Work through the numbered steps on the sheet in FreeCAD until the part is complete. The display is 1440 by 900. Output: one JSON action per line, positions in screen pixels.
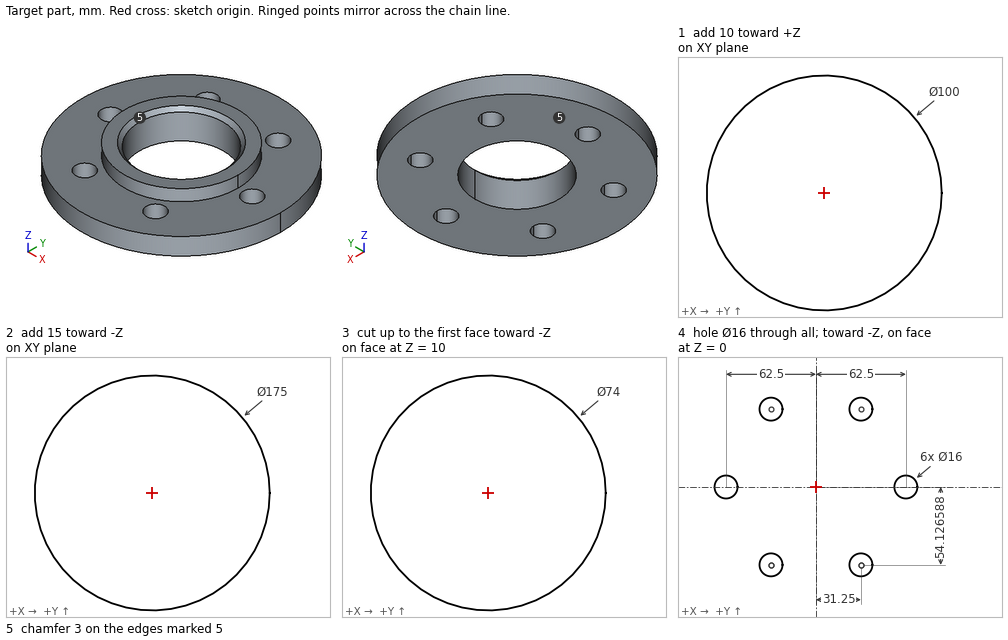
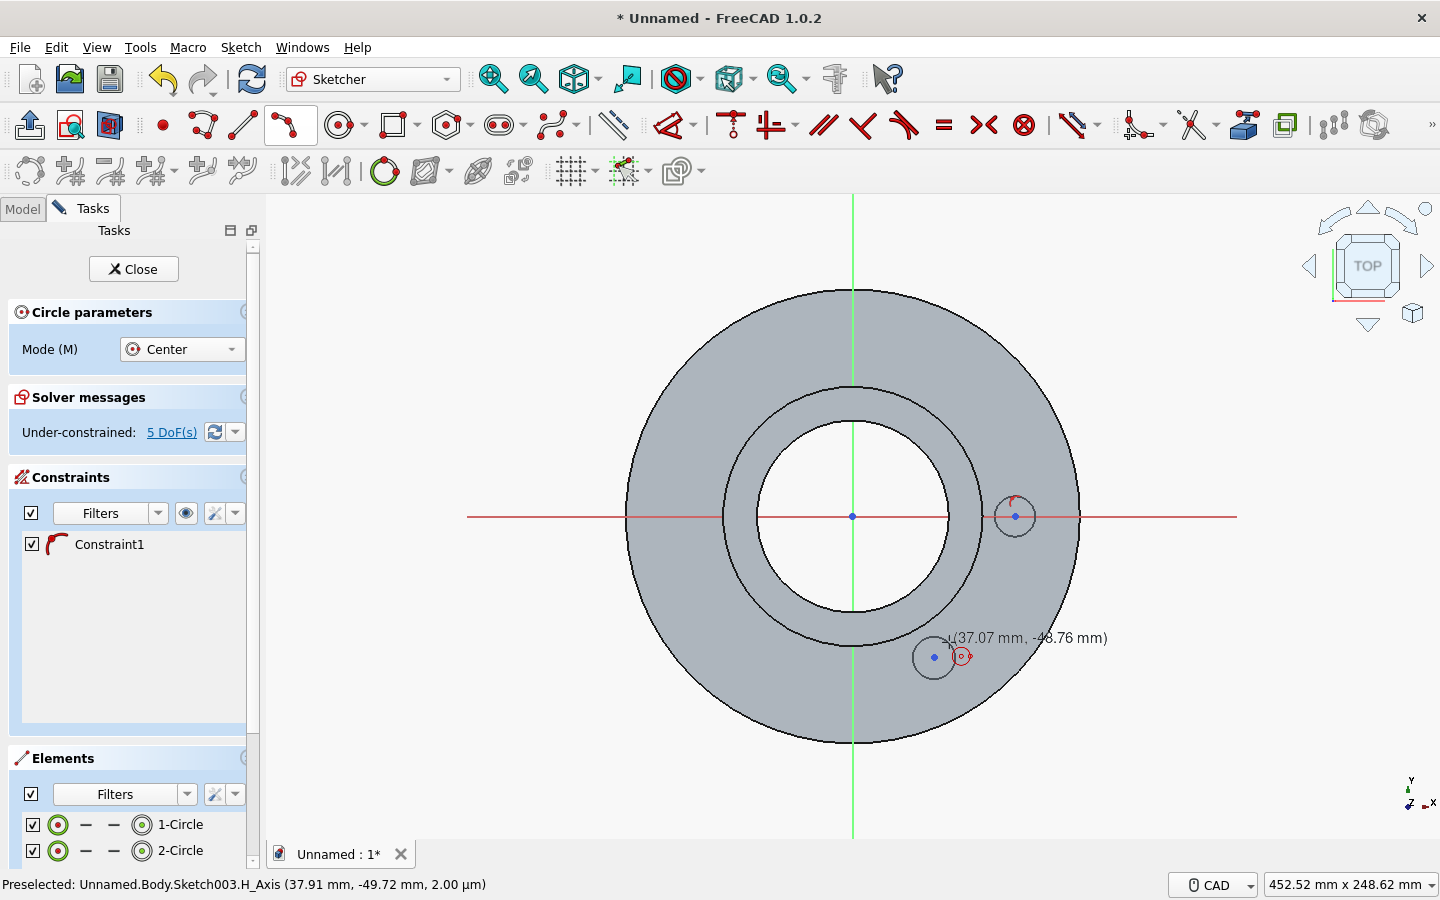
{"action": "left_click", "coordinate": [772, 657]}
{"action": "left_click", "coordinate": [786, 642]}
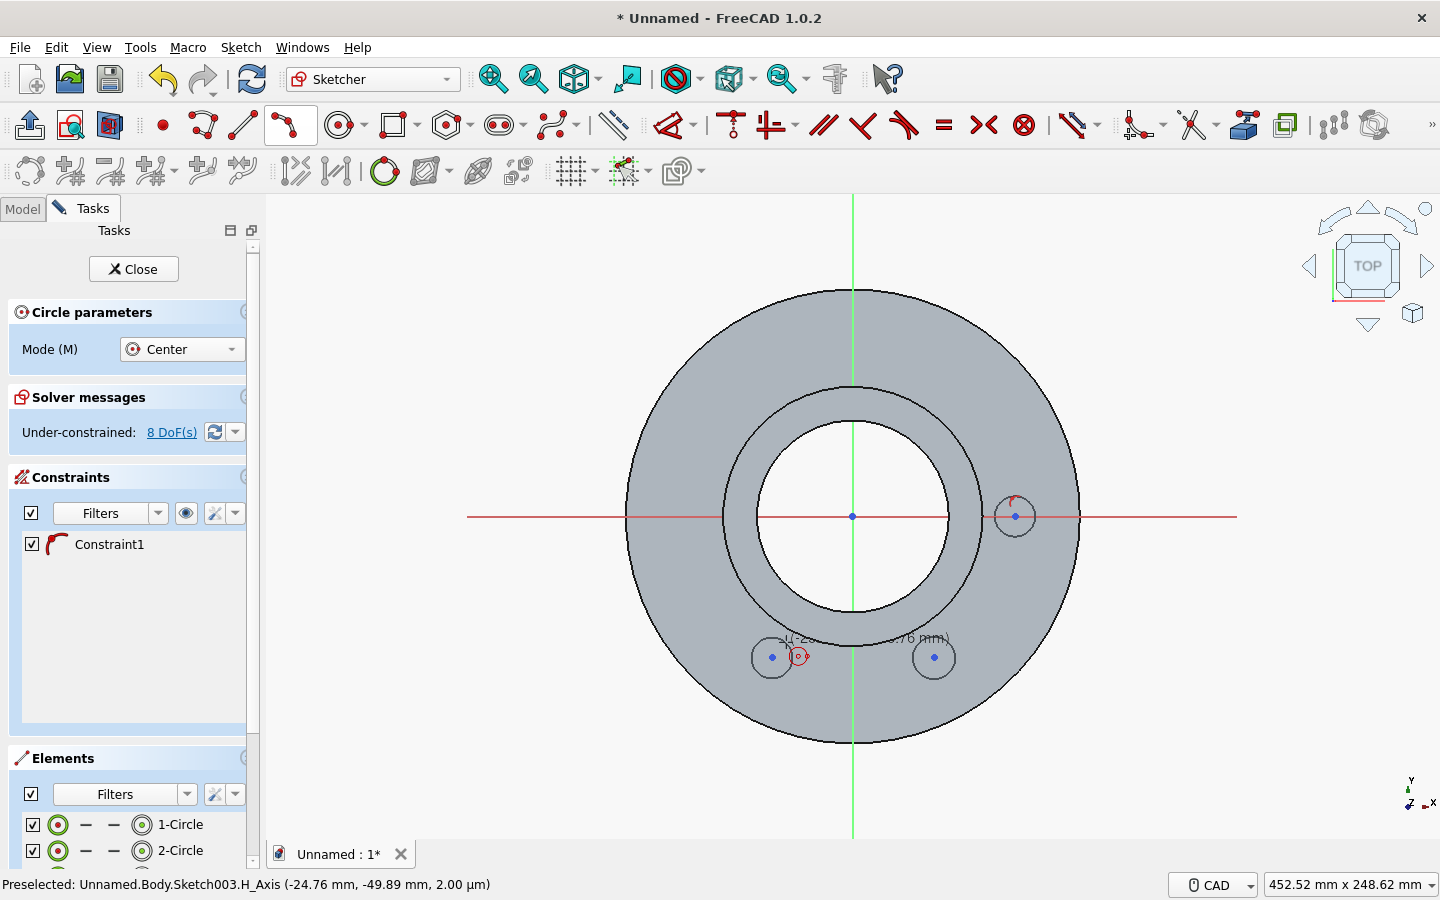
{"action": "left_click", "coordinate": [691, 516]}
{"action": "left_click", "coordinate": [705, 502]}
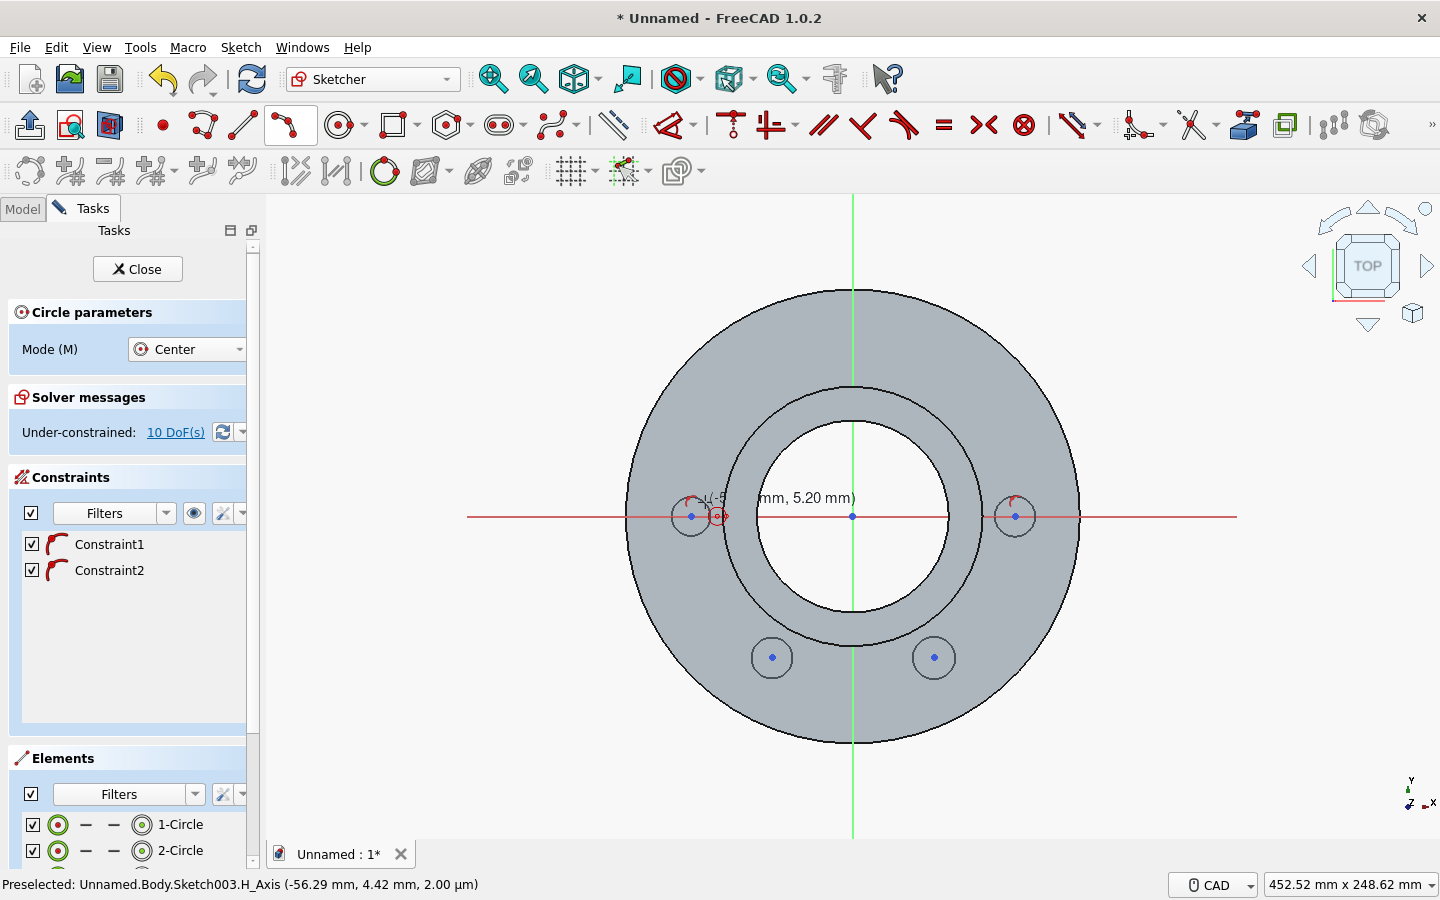
{"action": "left_click", "coordinate": [772, 376]}
{"action": "left_click", "coordinate": [786, 361]}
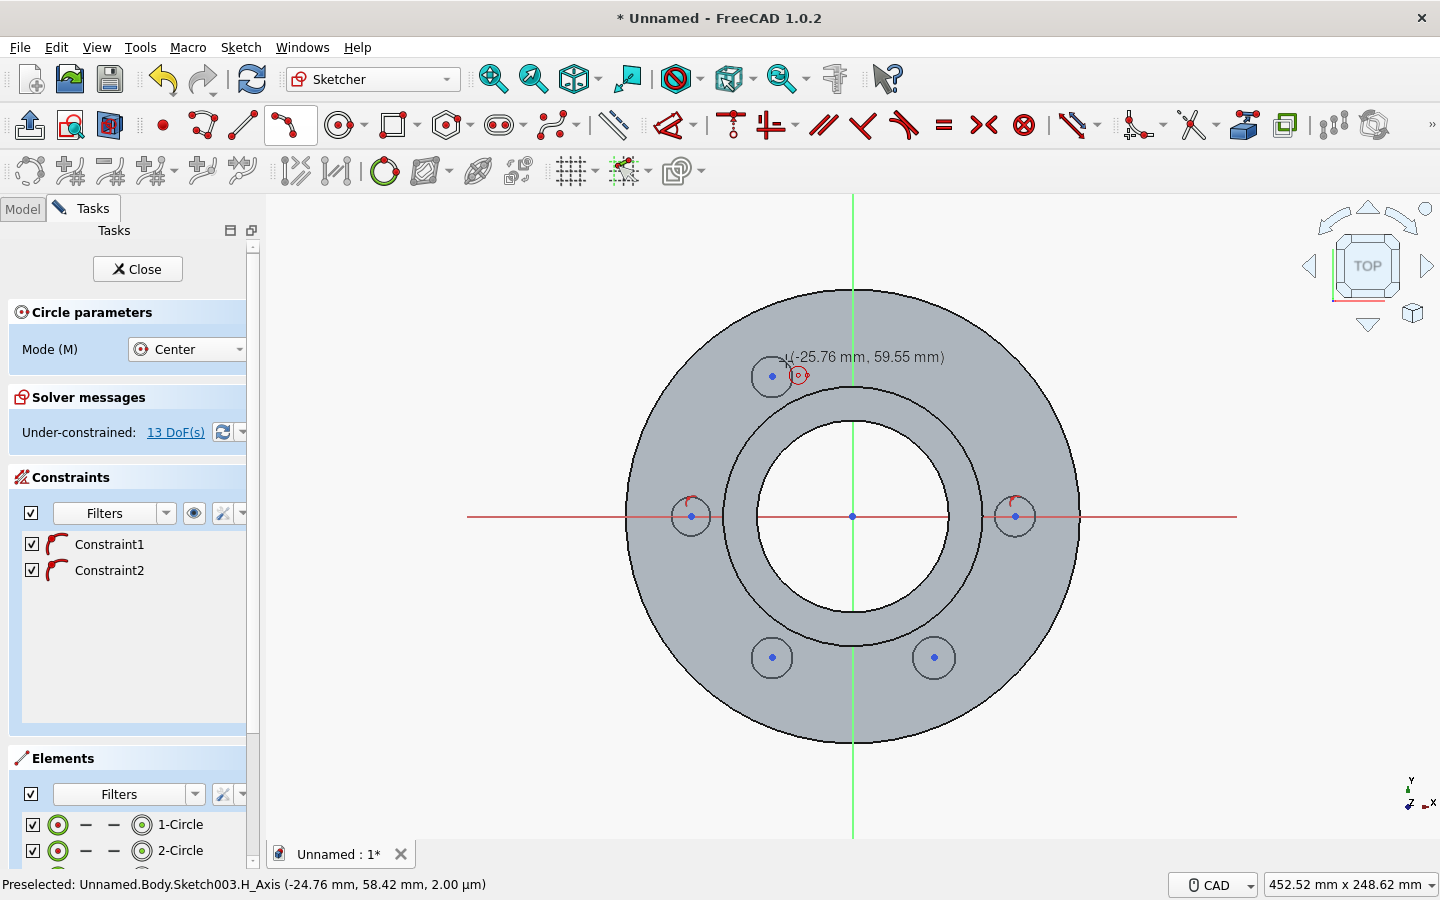
{"action": "left_click", "coordinate": [934, 376]}
{"action": "left_click", "coordinate": [949, 361]}
{"action": "key", "text": "Escape"}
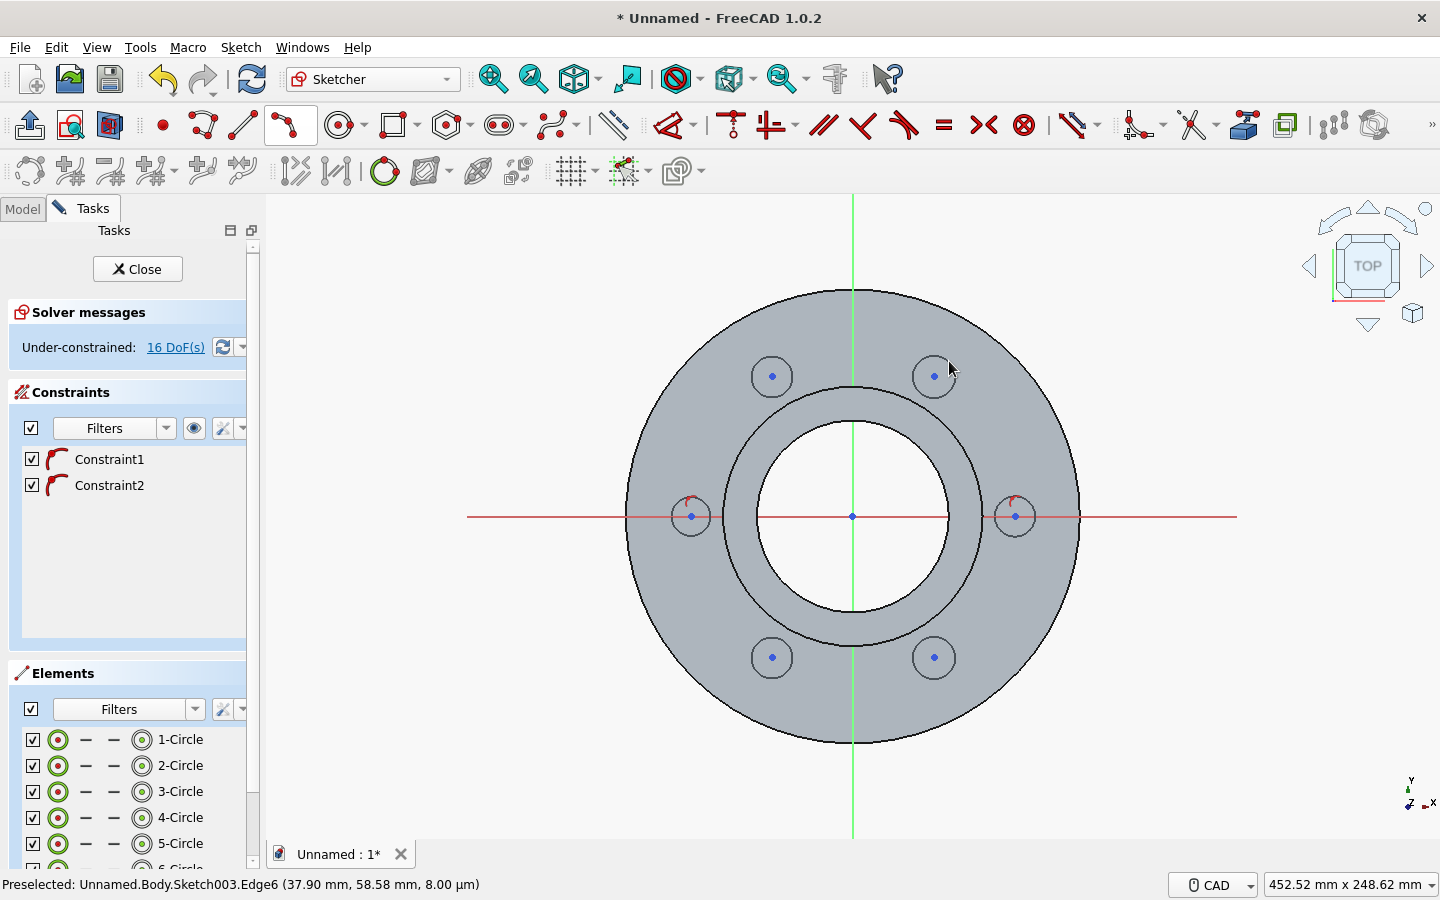
{"action": "left_click", "coordinate": [1029, 502]}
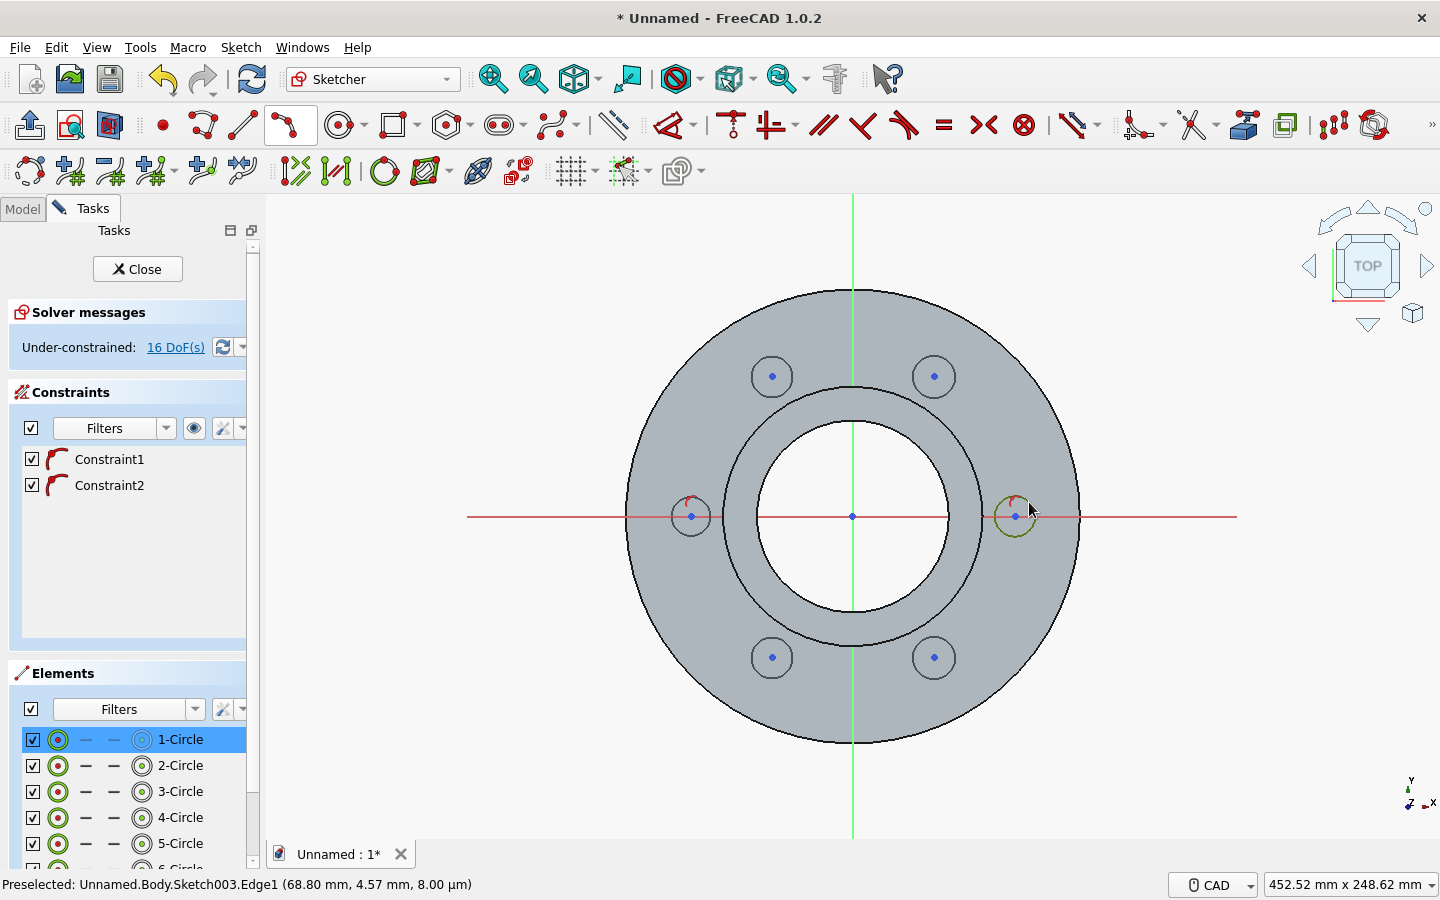
{"action": "left_click", "coordinate": [949, 643]}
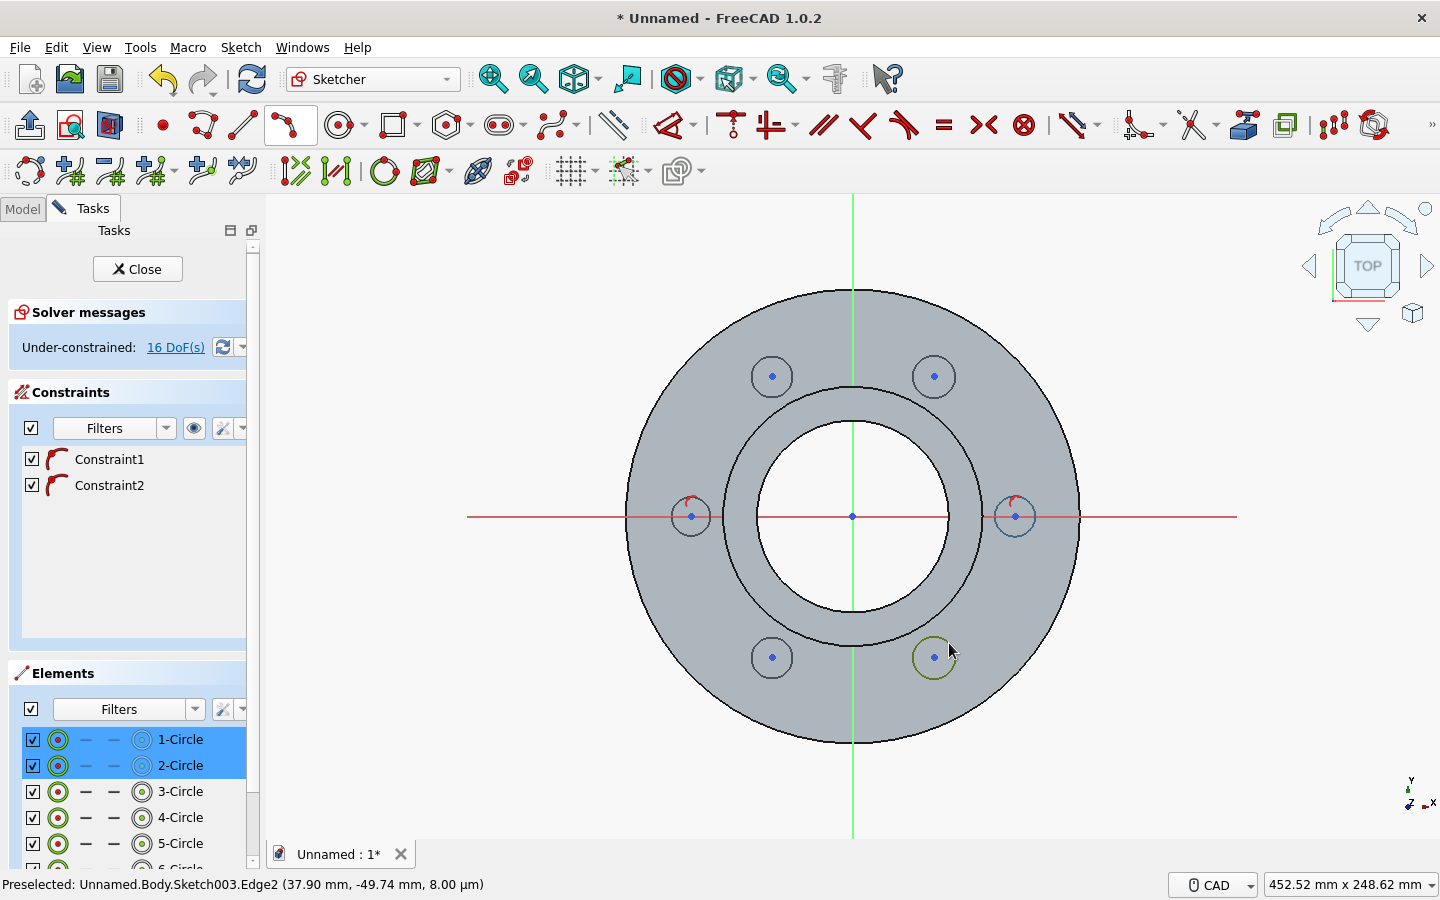
{"action": "left_click", "coordinate": [786, 643]}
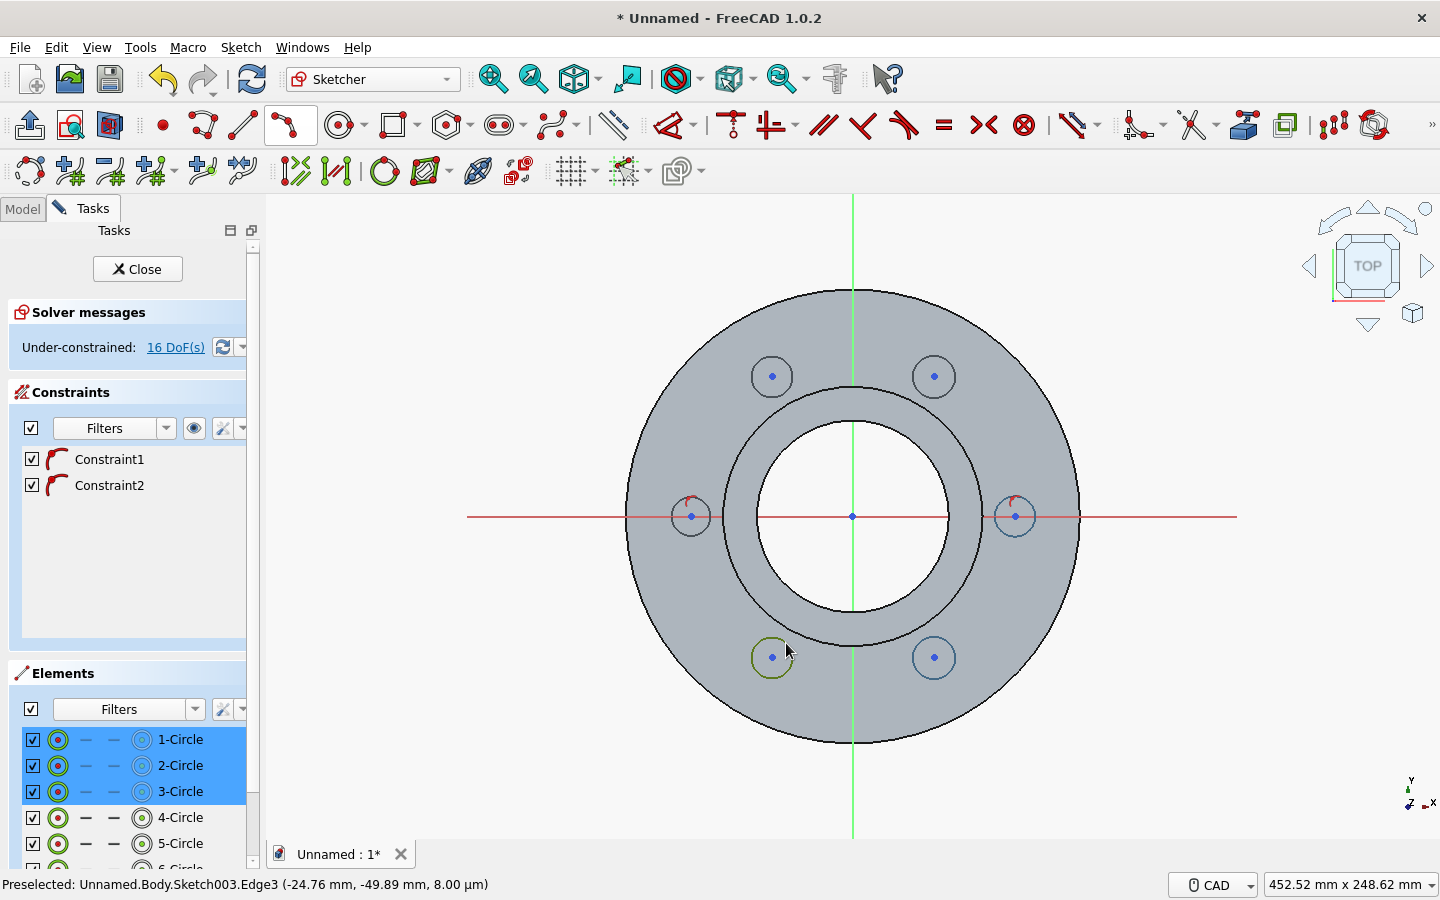
{"action": "left_click", "coordinate": [705, 503]}